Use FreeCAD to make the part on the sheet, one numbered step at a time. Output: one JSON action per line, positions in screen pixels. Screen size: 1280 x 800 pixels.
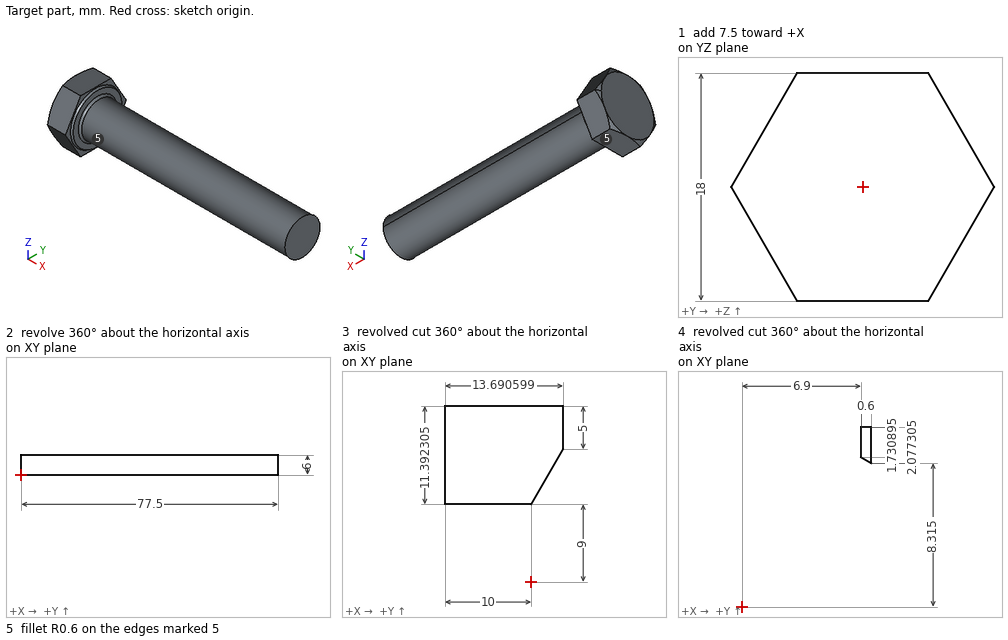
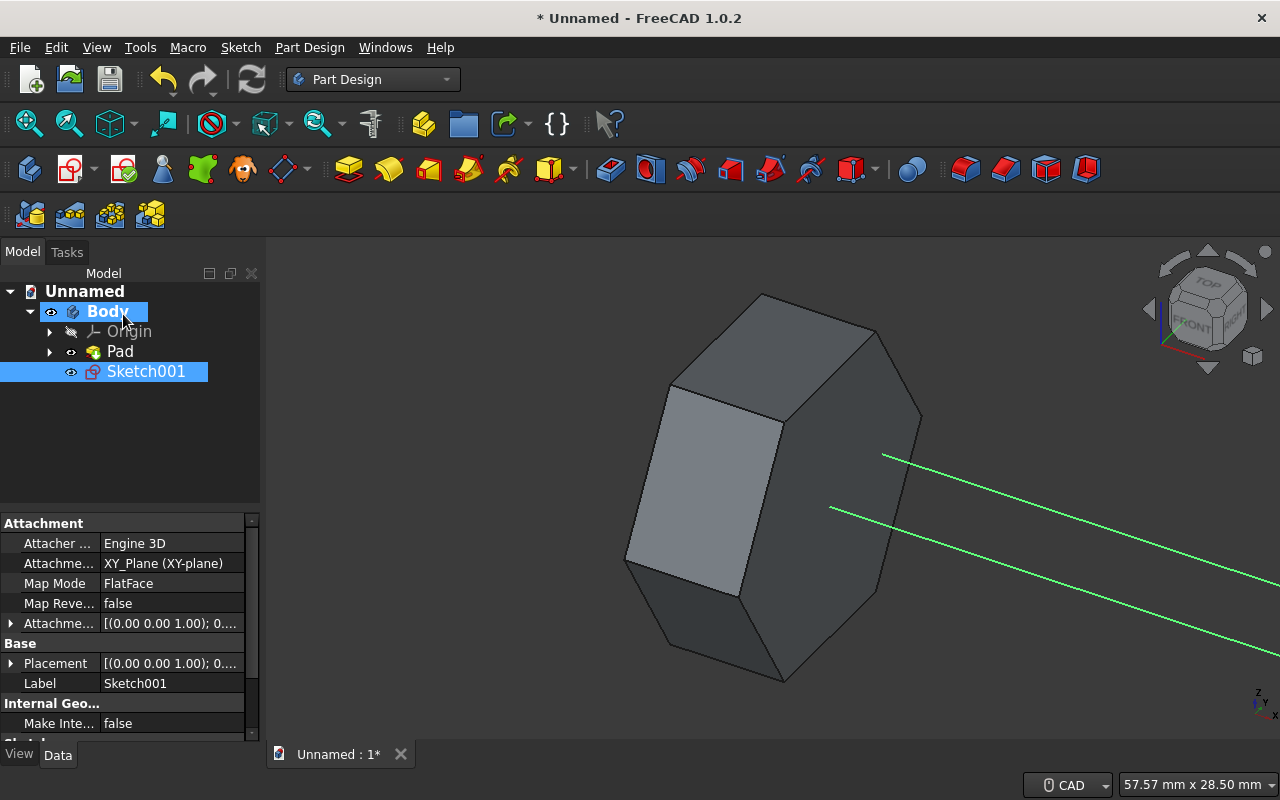
{"action": "left_click", "coordinate": [390, 170]}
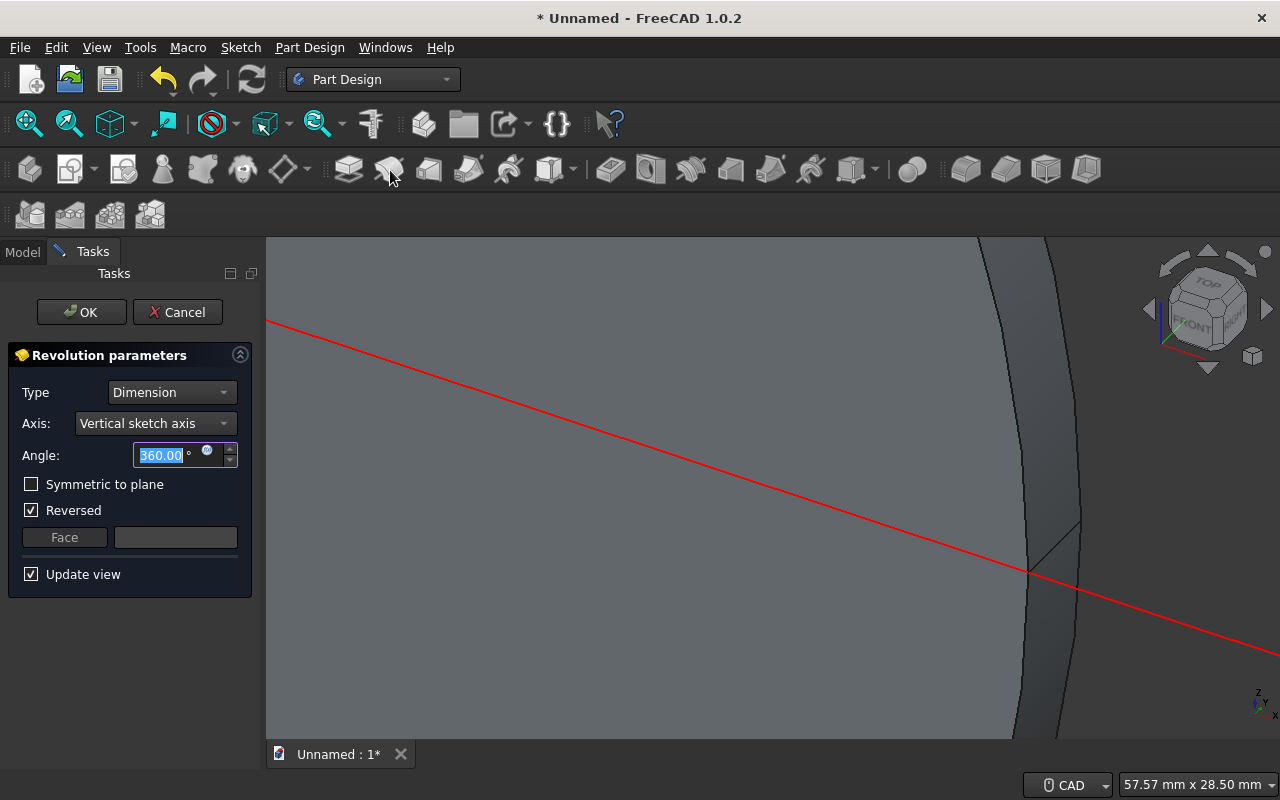
{"action": "left_click", "coordinate": [156, 424]}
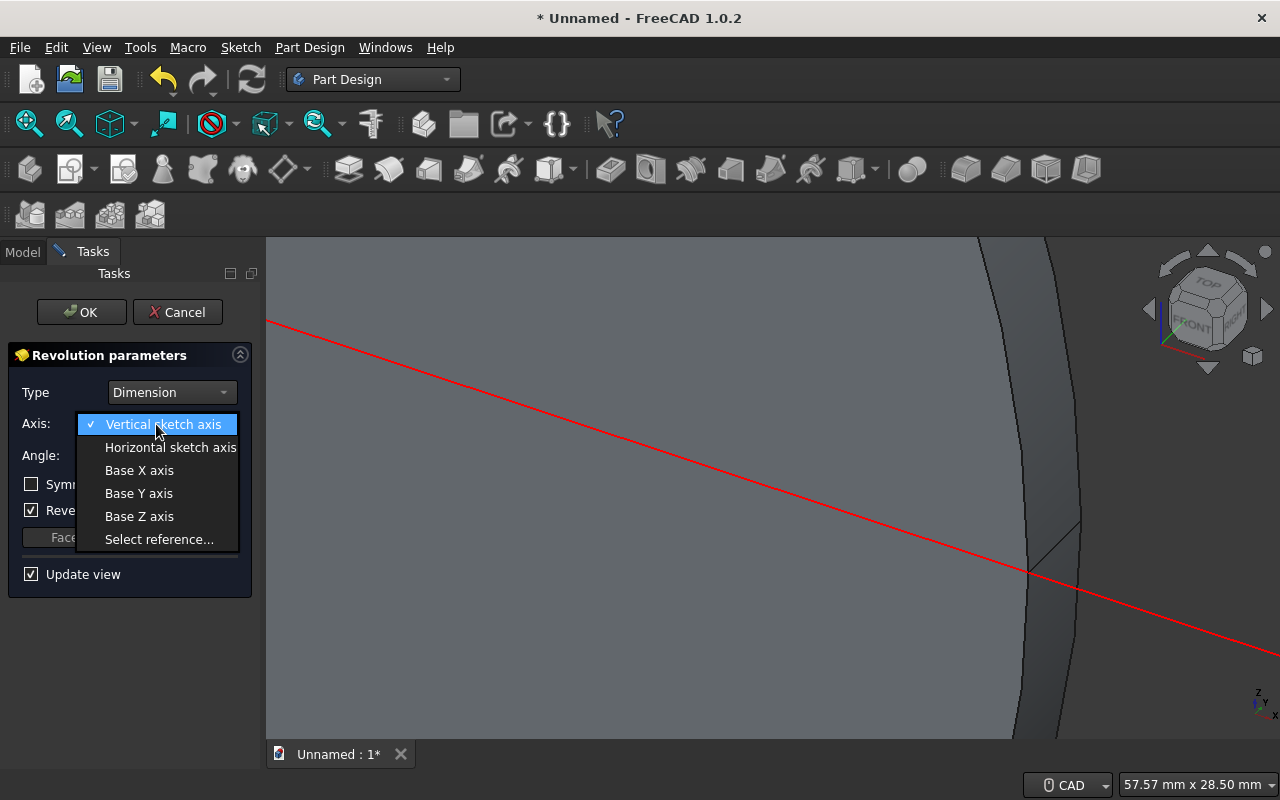
{"action": "left_click", "coordinate": [156, 448]}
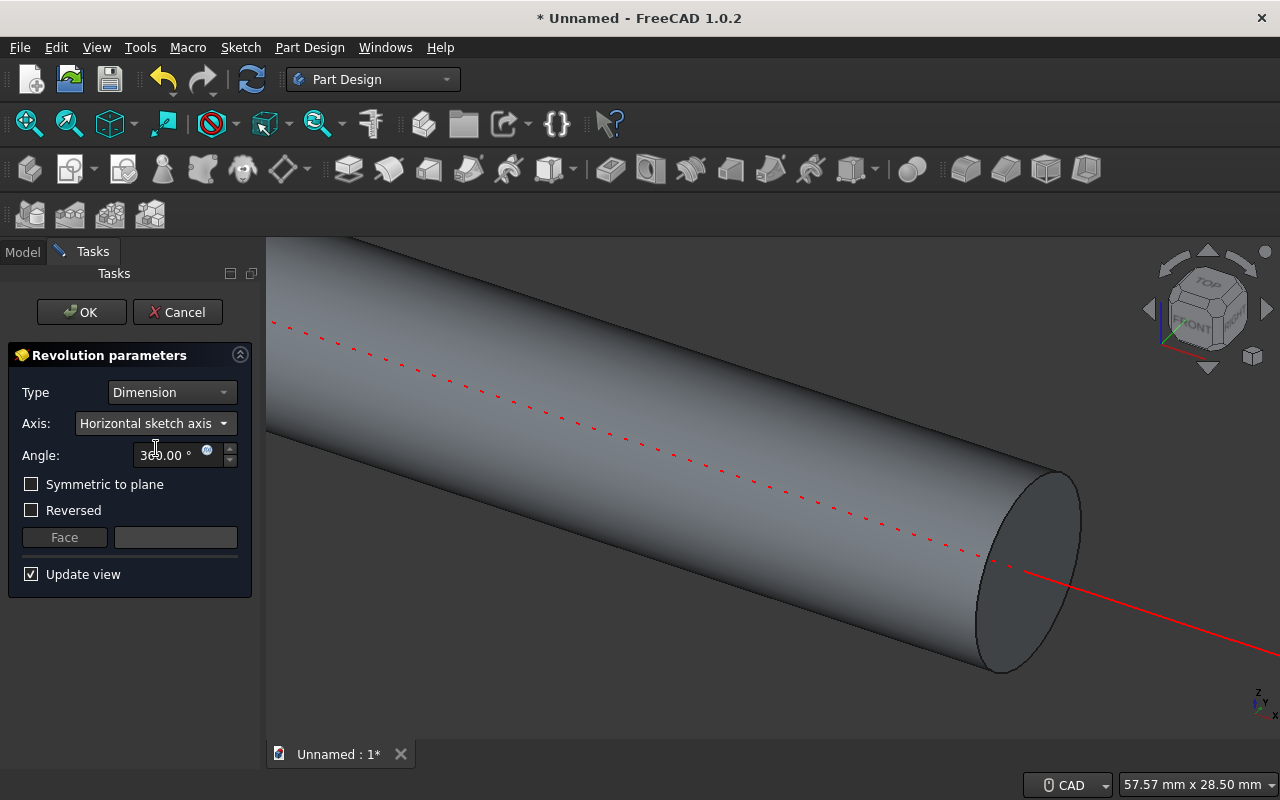
{"action": "left_click", "coordinate": [82, 312]}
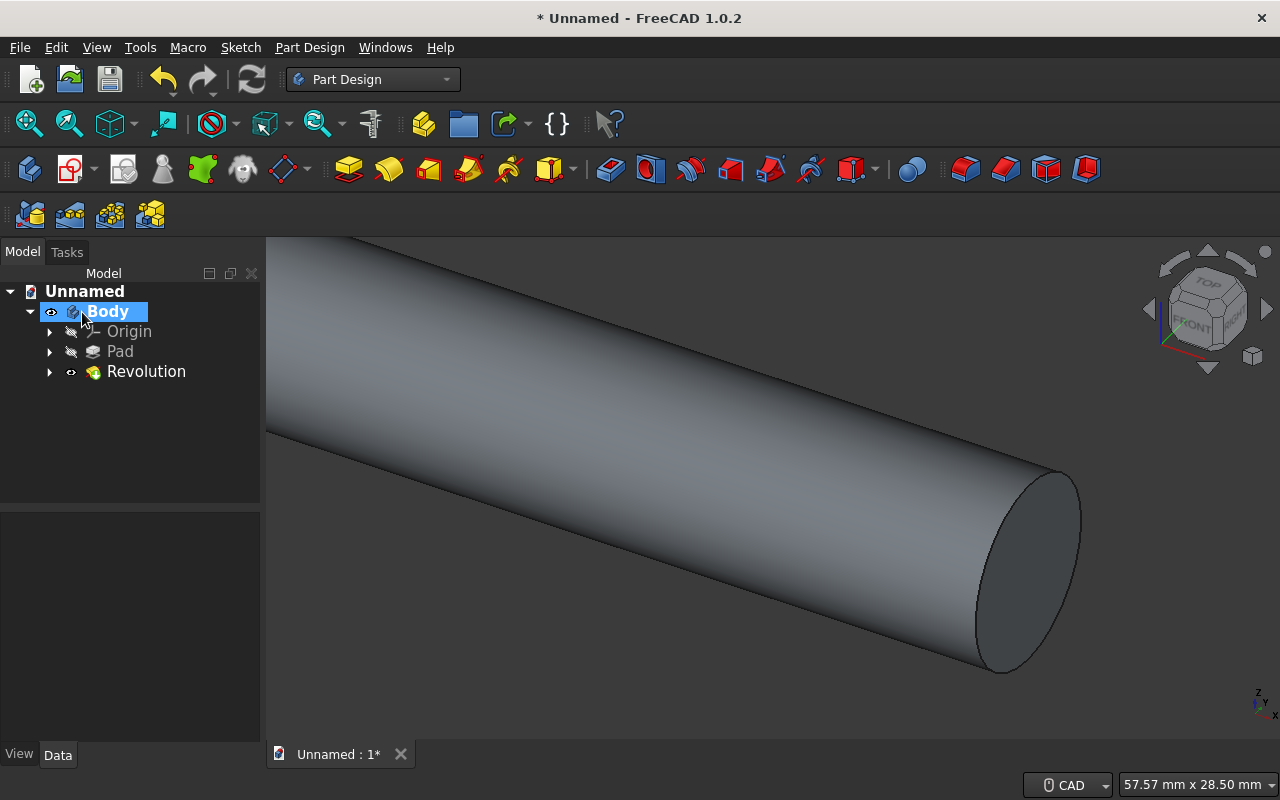
{"action": "left_click", "coordinate": [30, 124]}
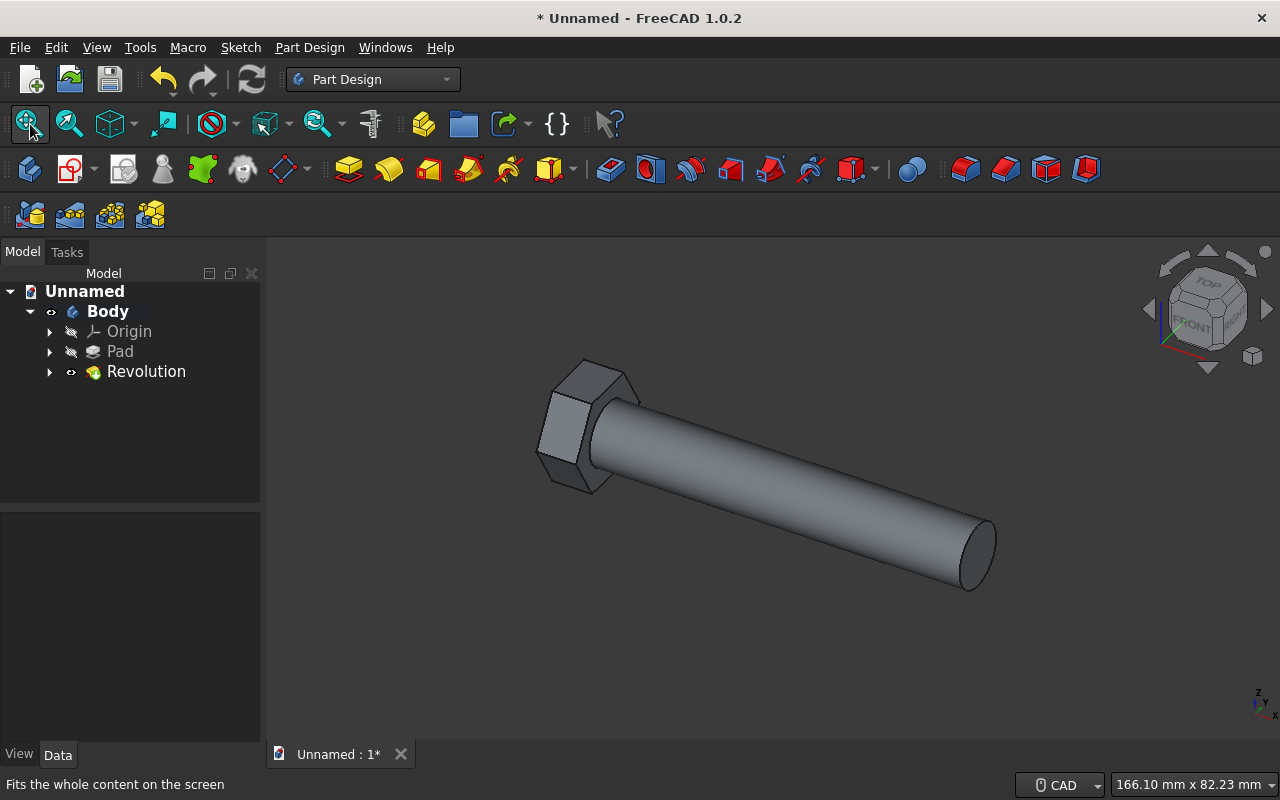
{"action": "left_click", "coordinate": [70, 170]}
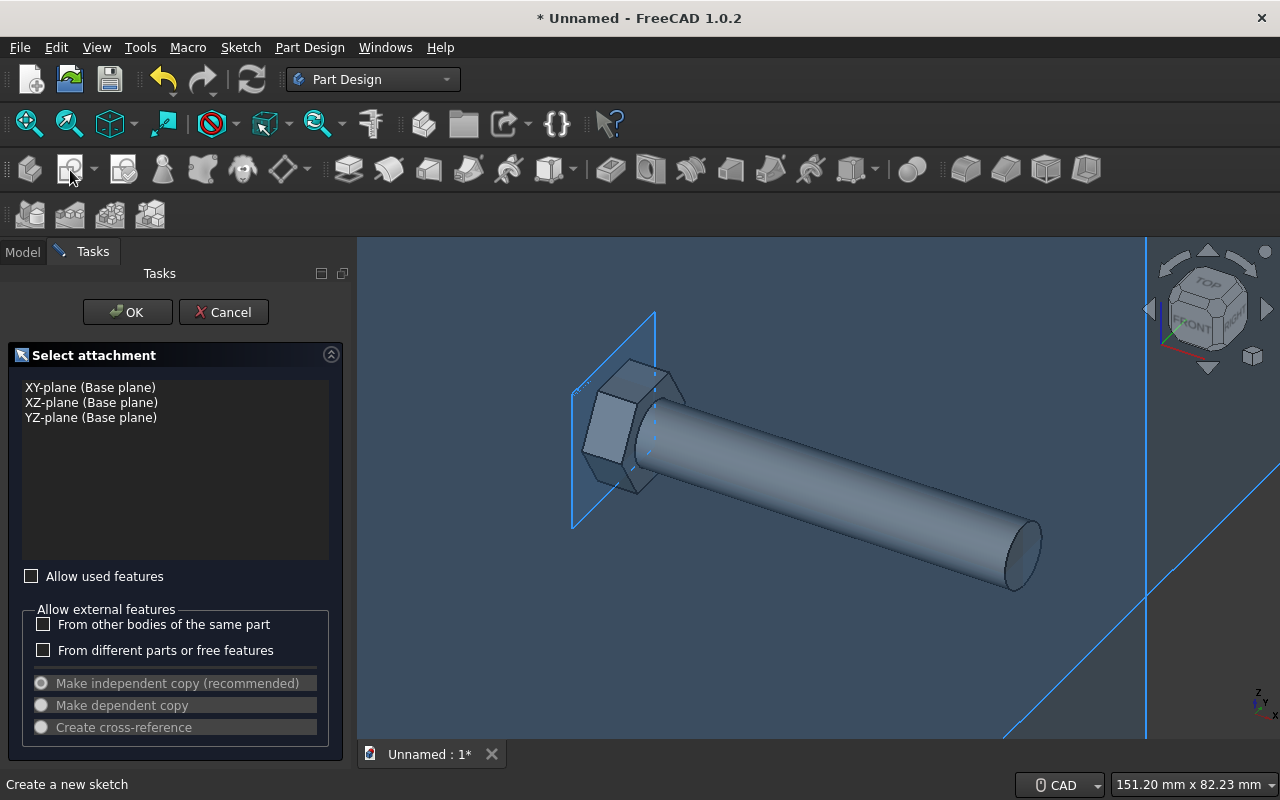
{"action": "left_click", "coordinate": [82, 388]}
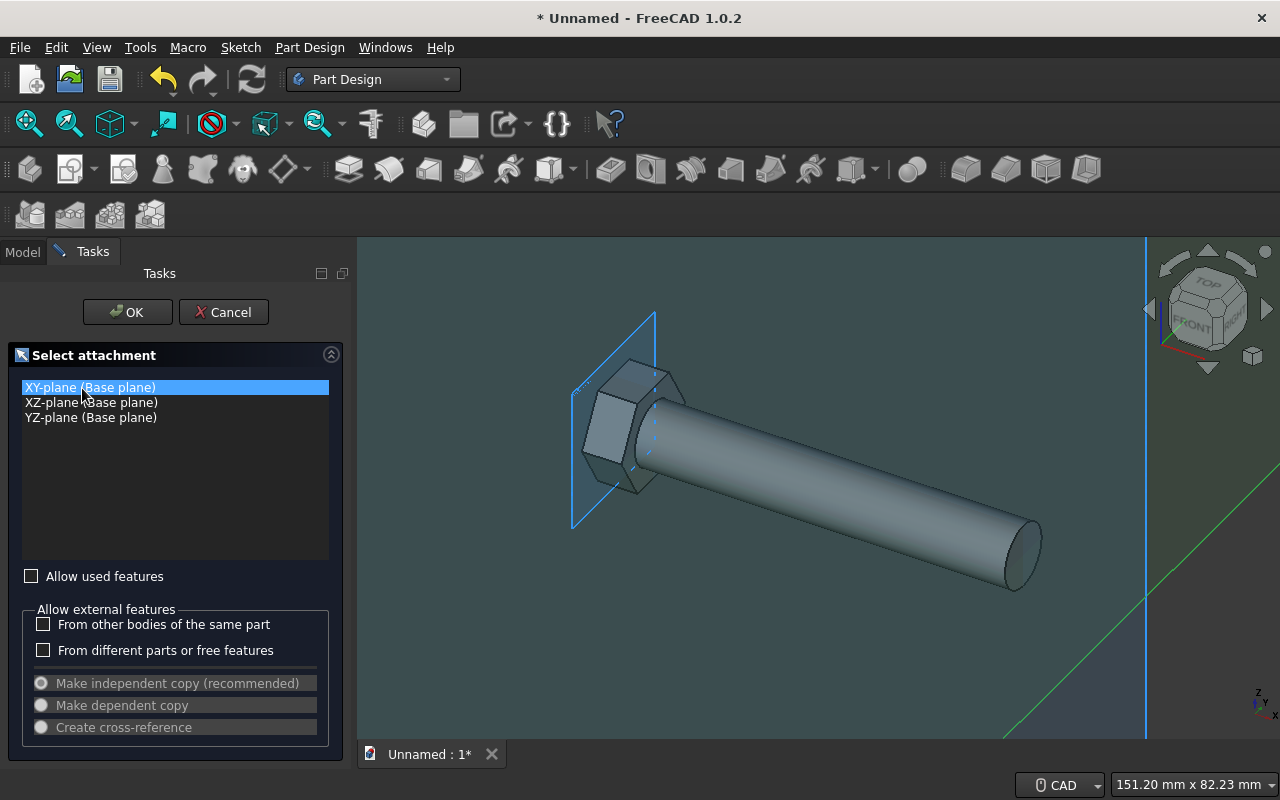
{"action": "left_click", "coordinate": [128, 312]}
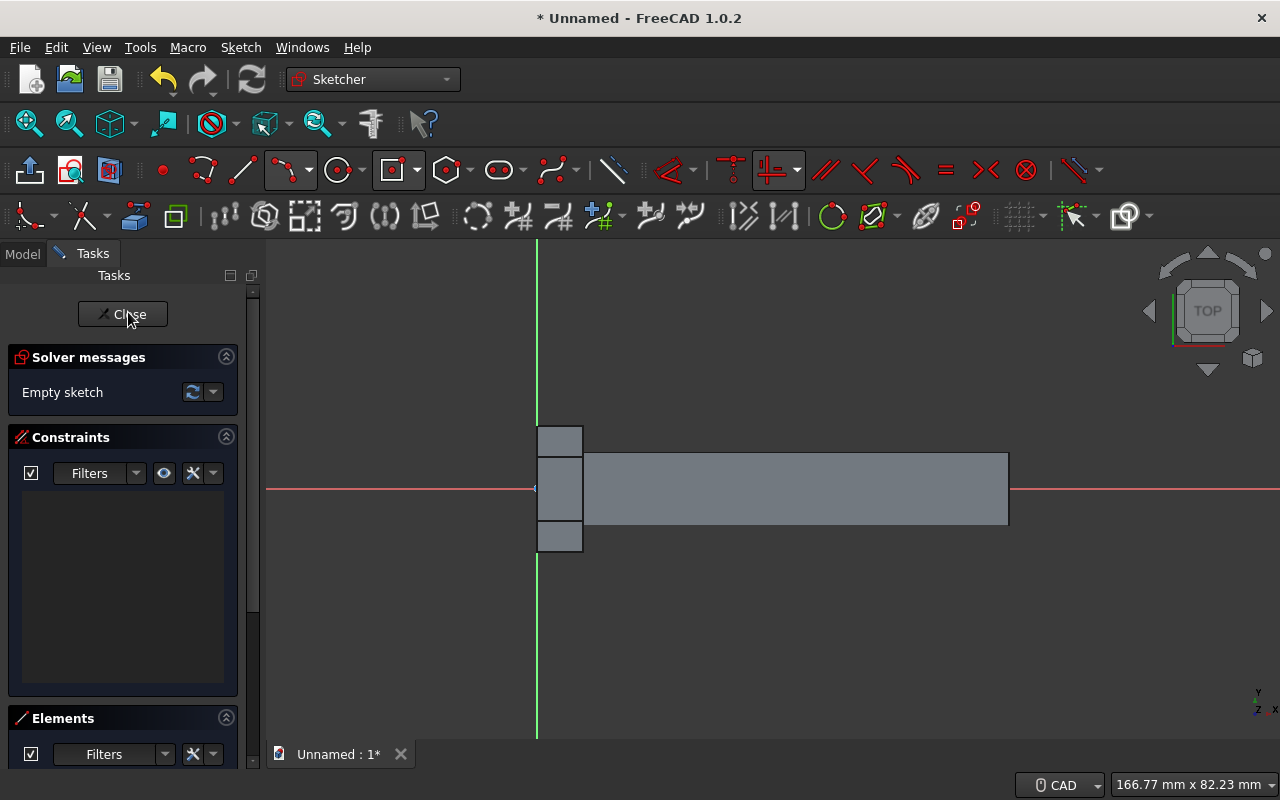
{"action": "left_click", "coordinate": [110, 170]}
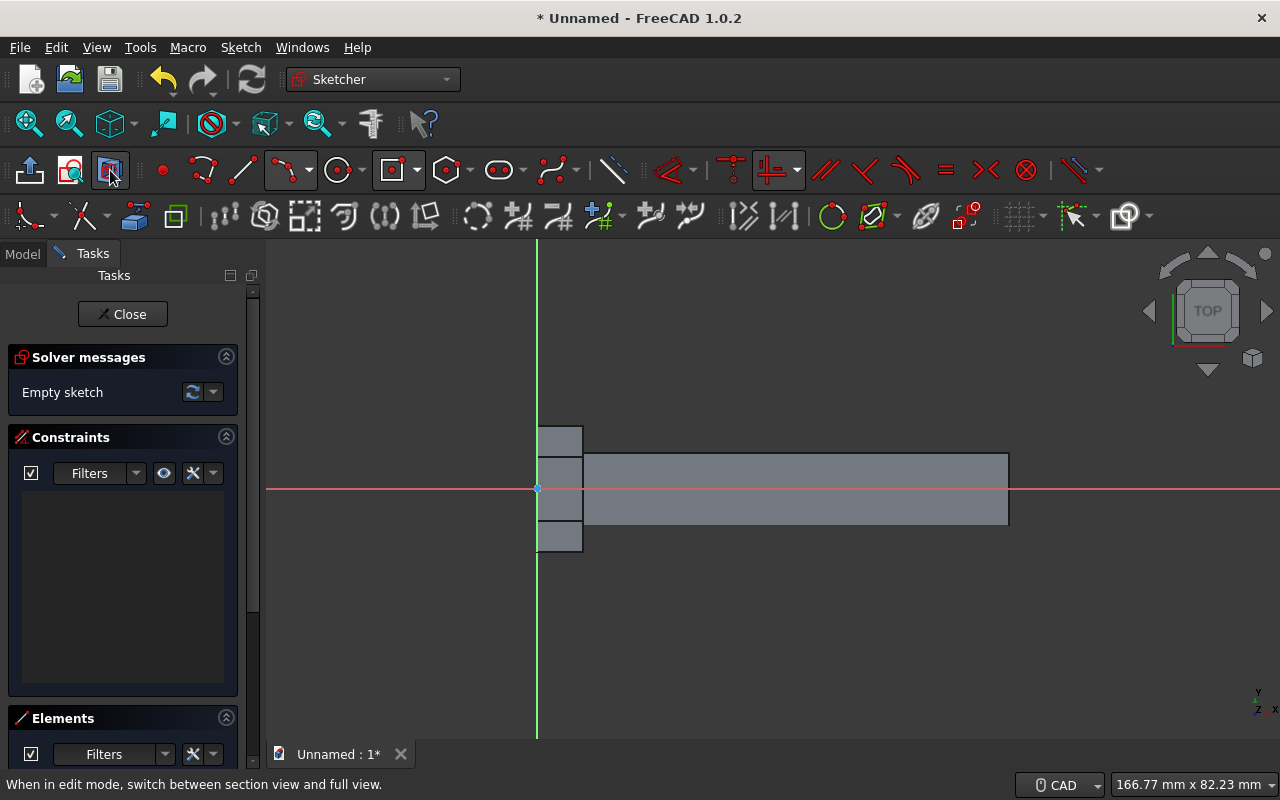
{"action": "scroll", "coordinate": [410, 391], "scroll_direction": "up", "scroll_amount": 5}